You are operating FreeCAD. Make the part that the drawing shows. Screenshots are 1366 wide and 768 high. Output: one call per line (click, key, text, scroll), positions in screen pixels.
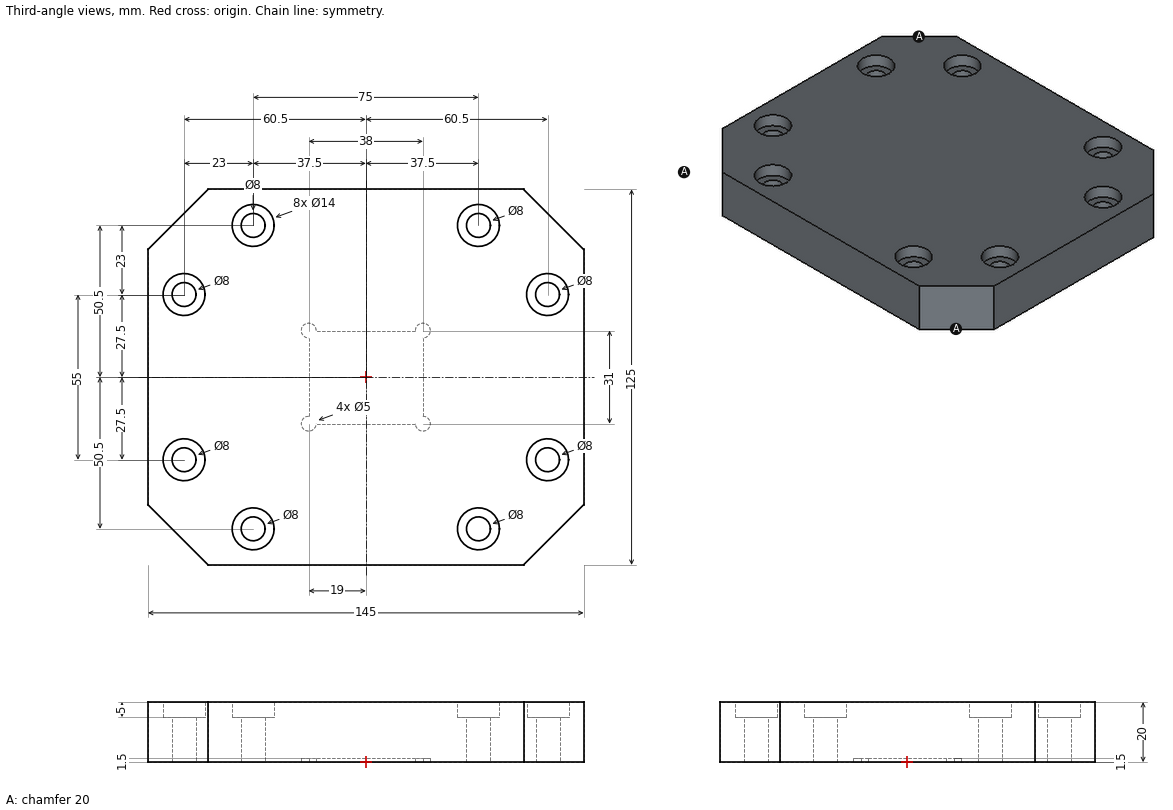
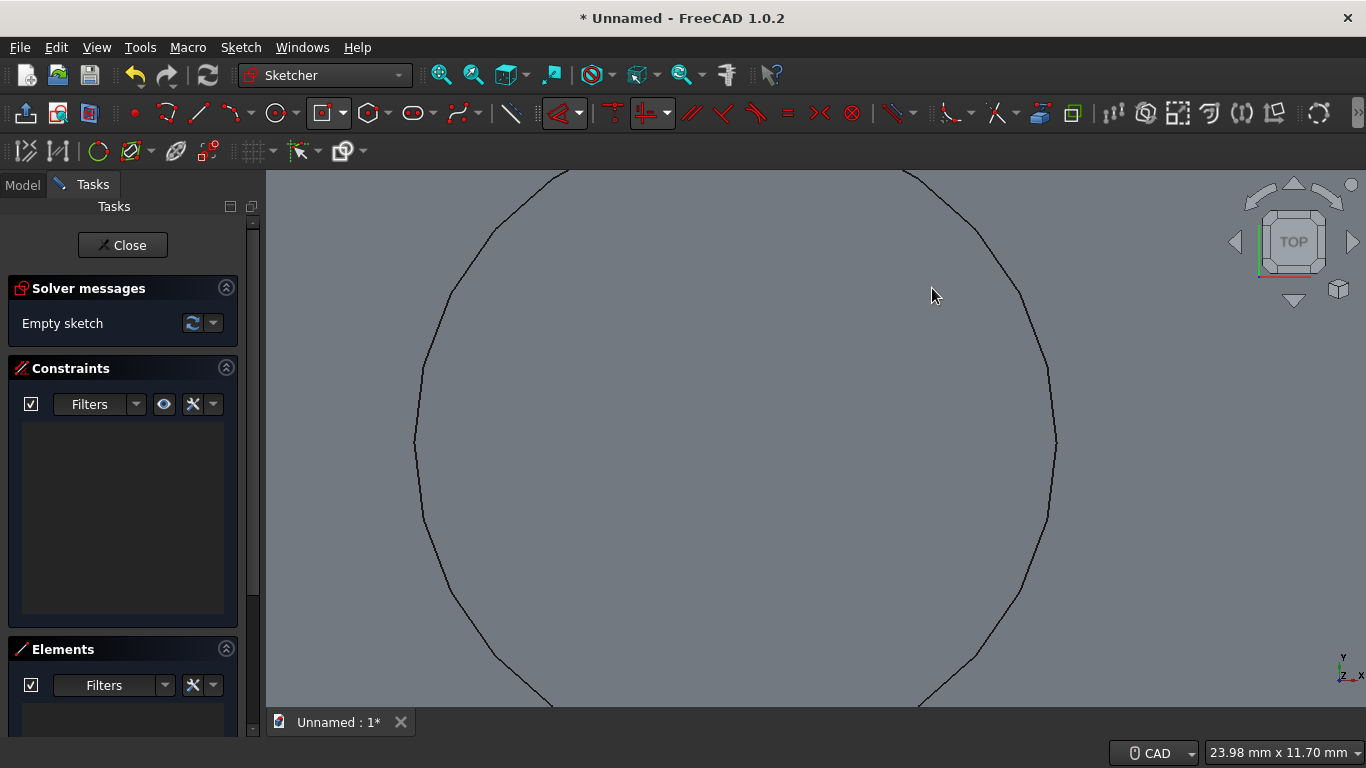
click(276, 114)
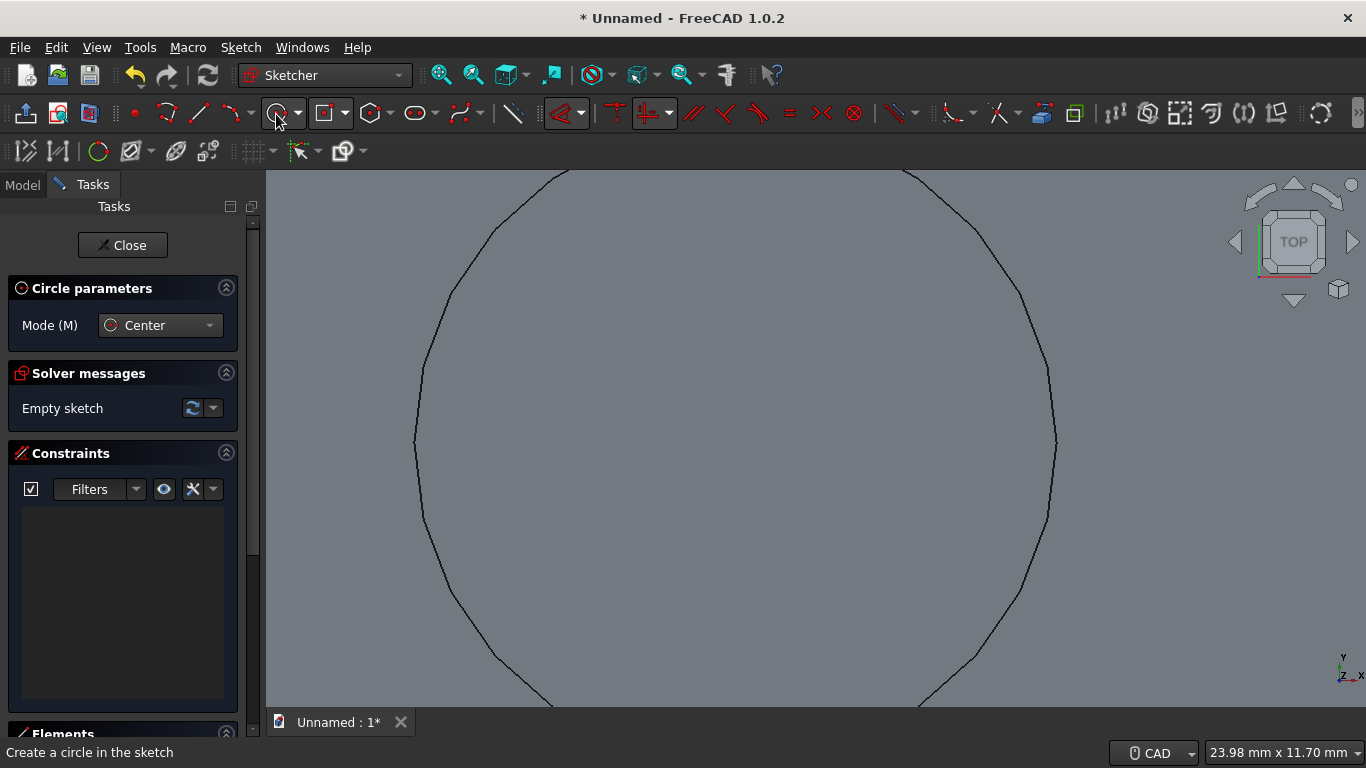
click(735, 443)
click(865, 313)
key(Escape)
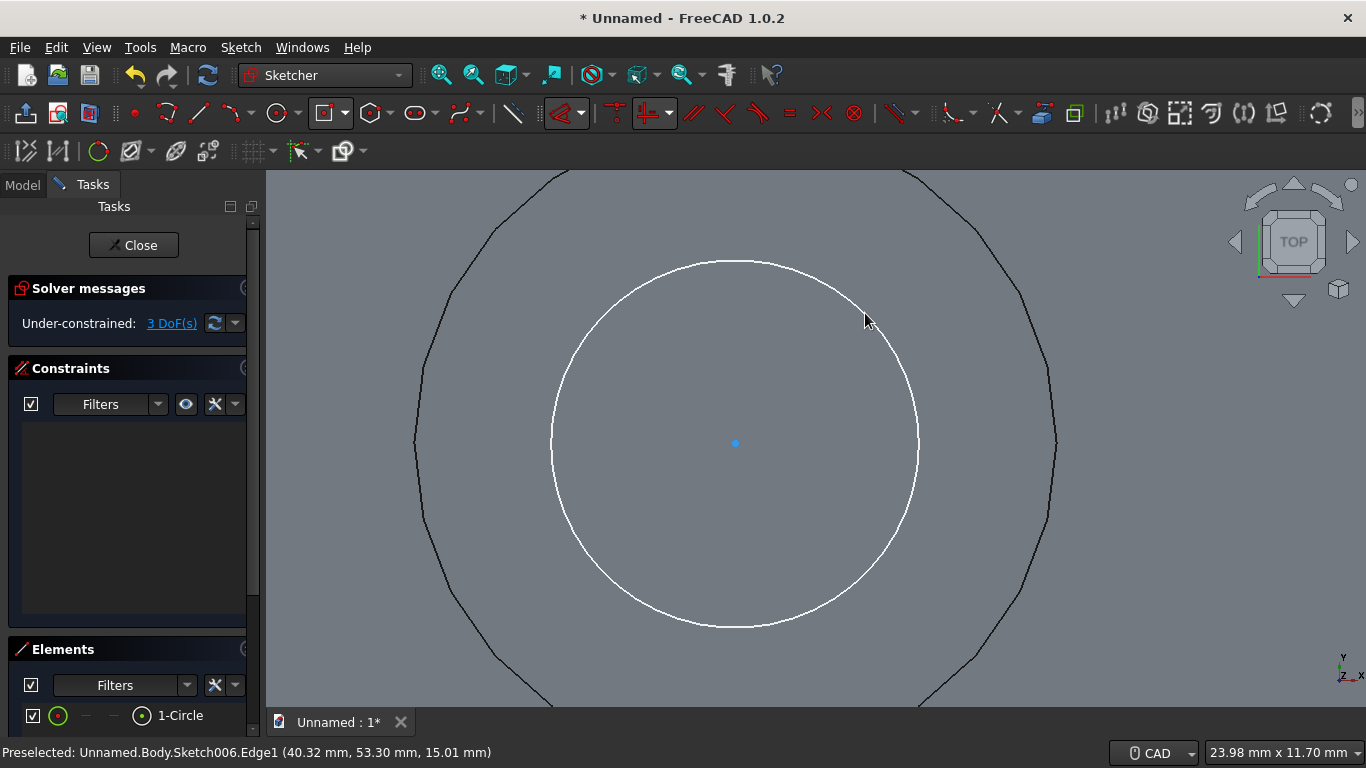
click(865, 314)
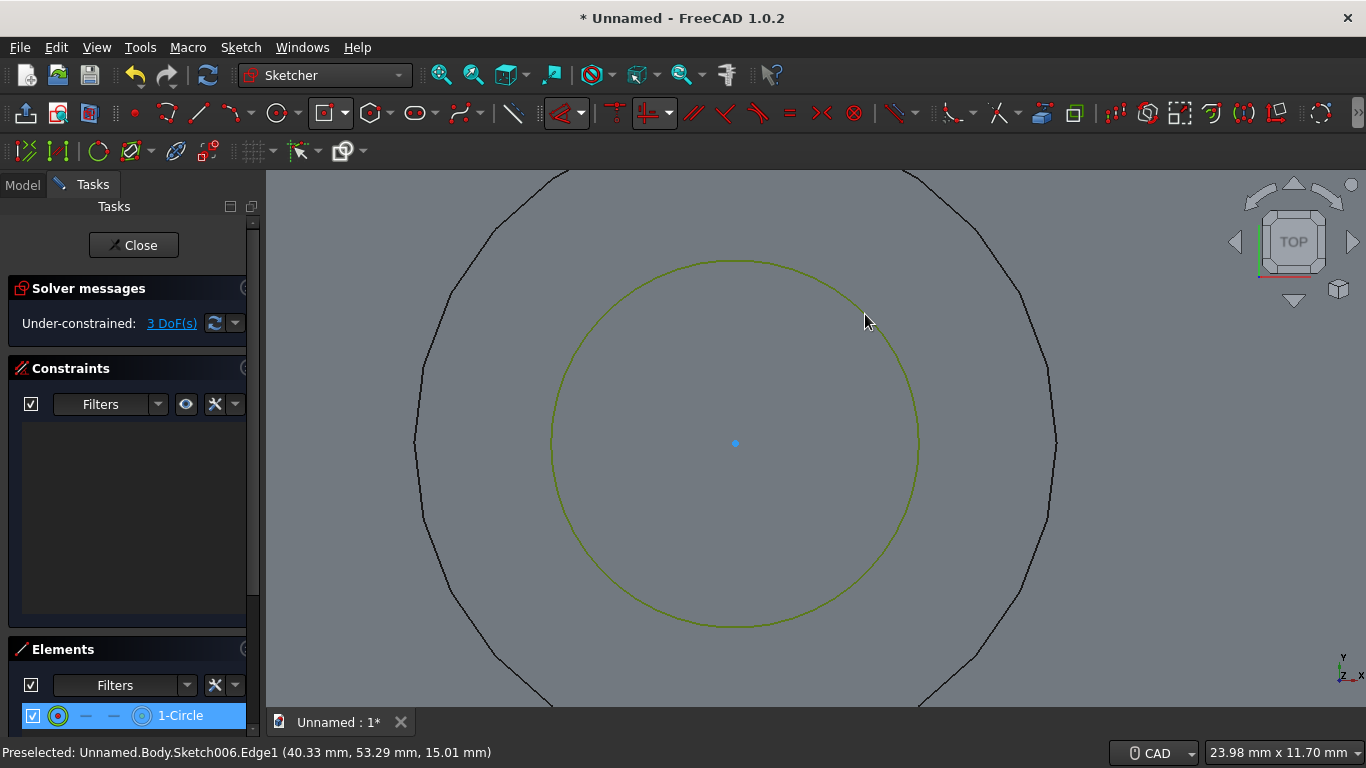
key(k)
key(o)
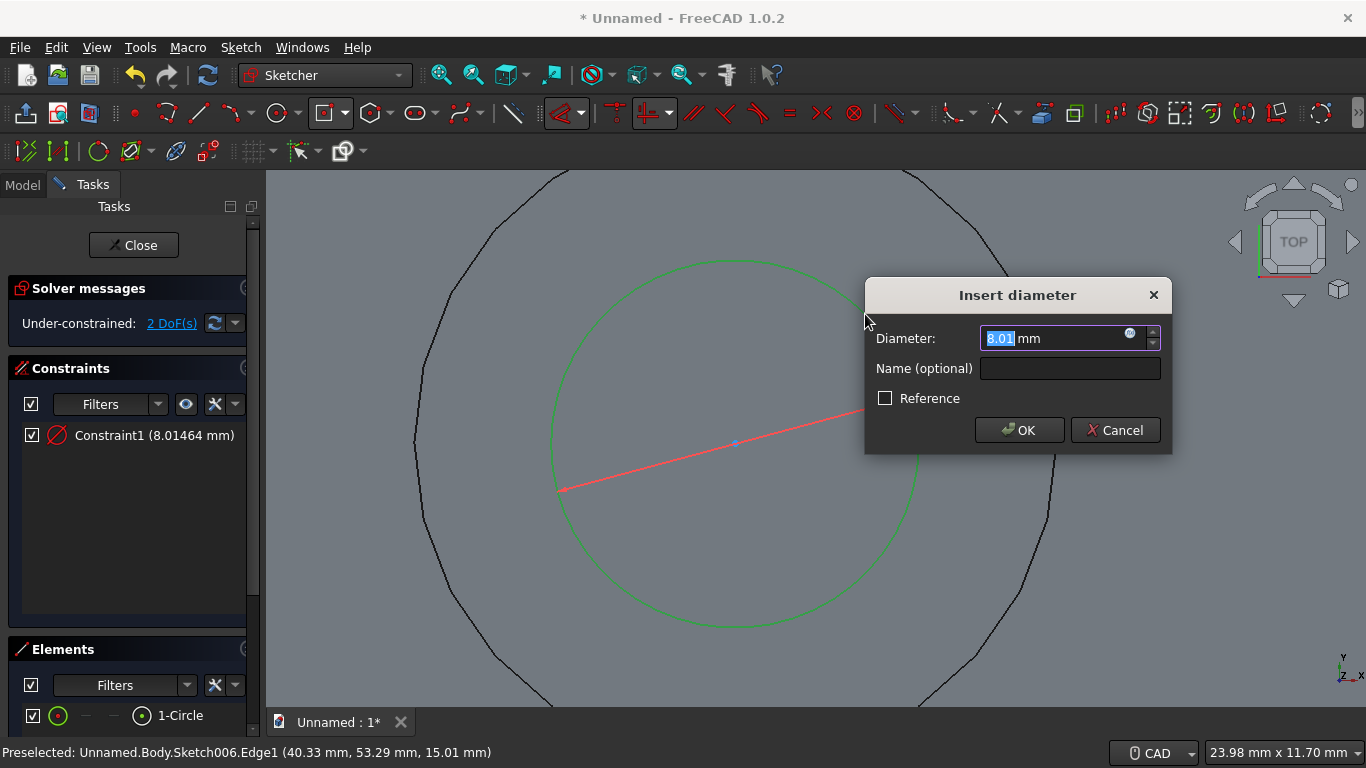
text(8)
key(Return)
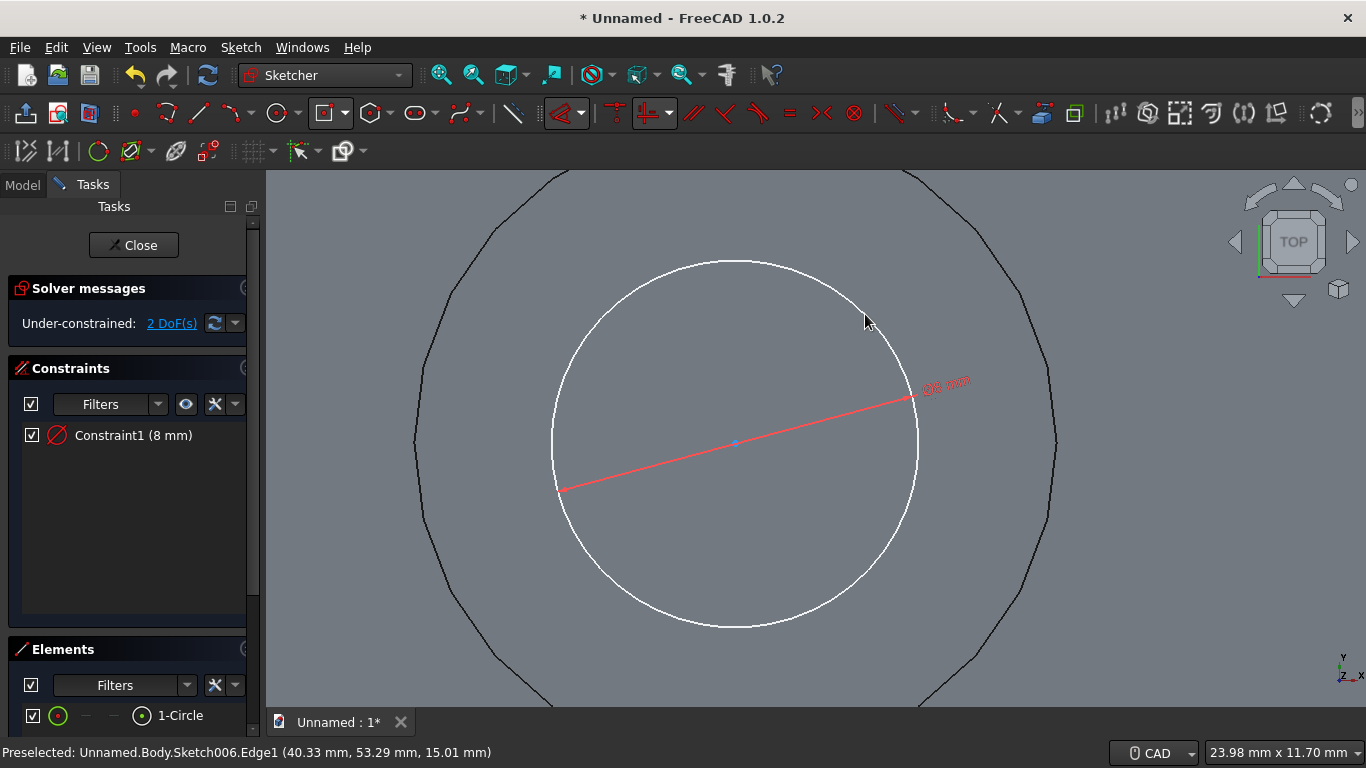
click(735, 444)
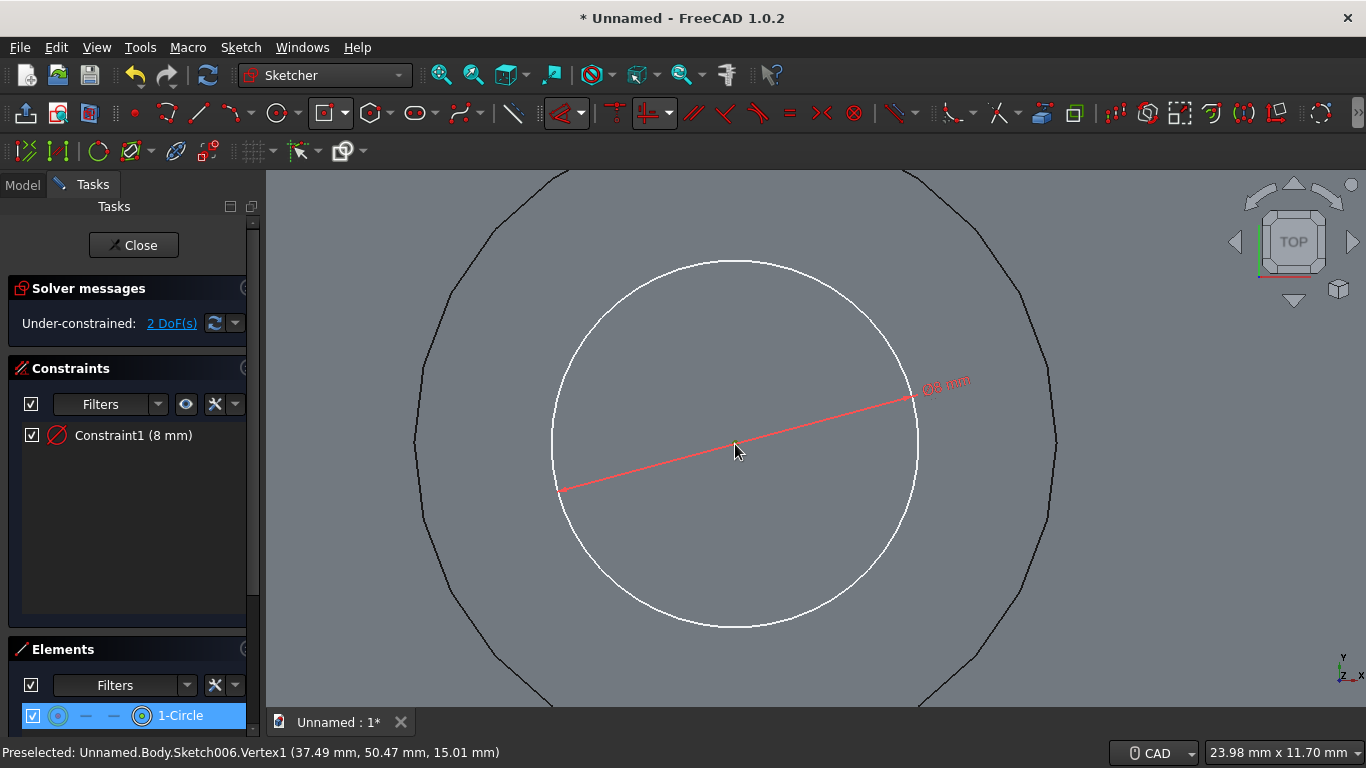
key(l)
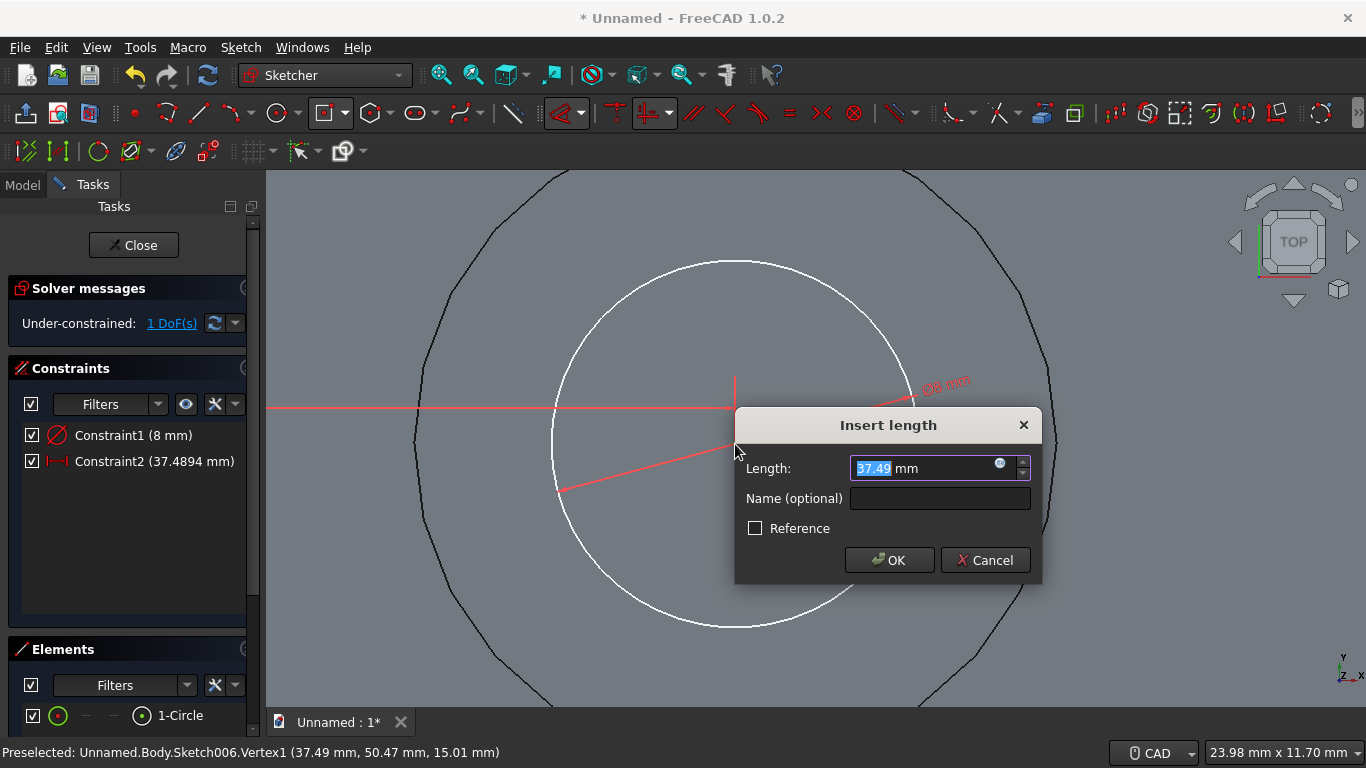
text(37.5)
key(Return)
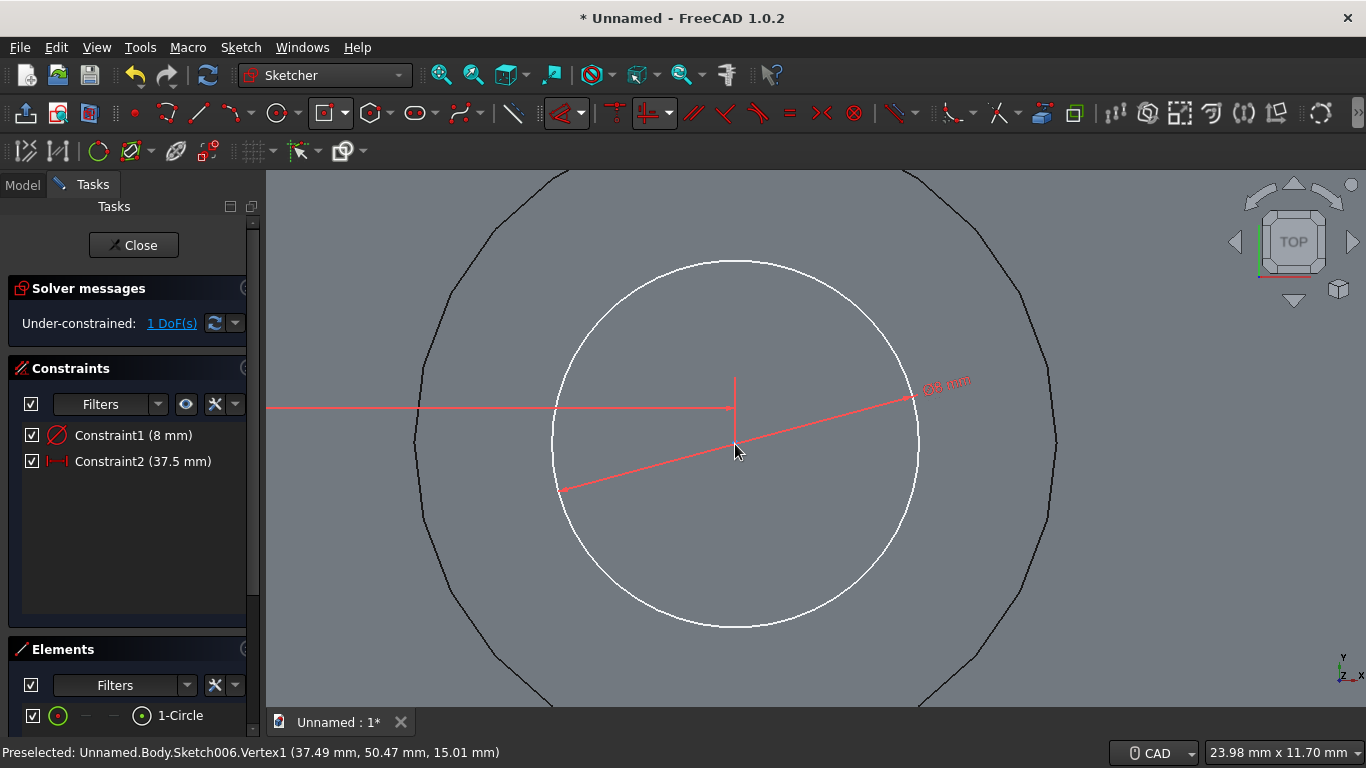
click(735, 444)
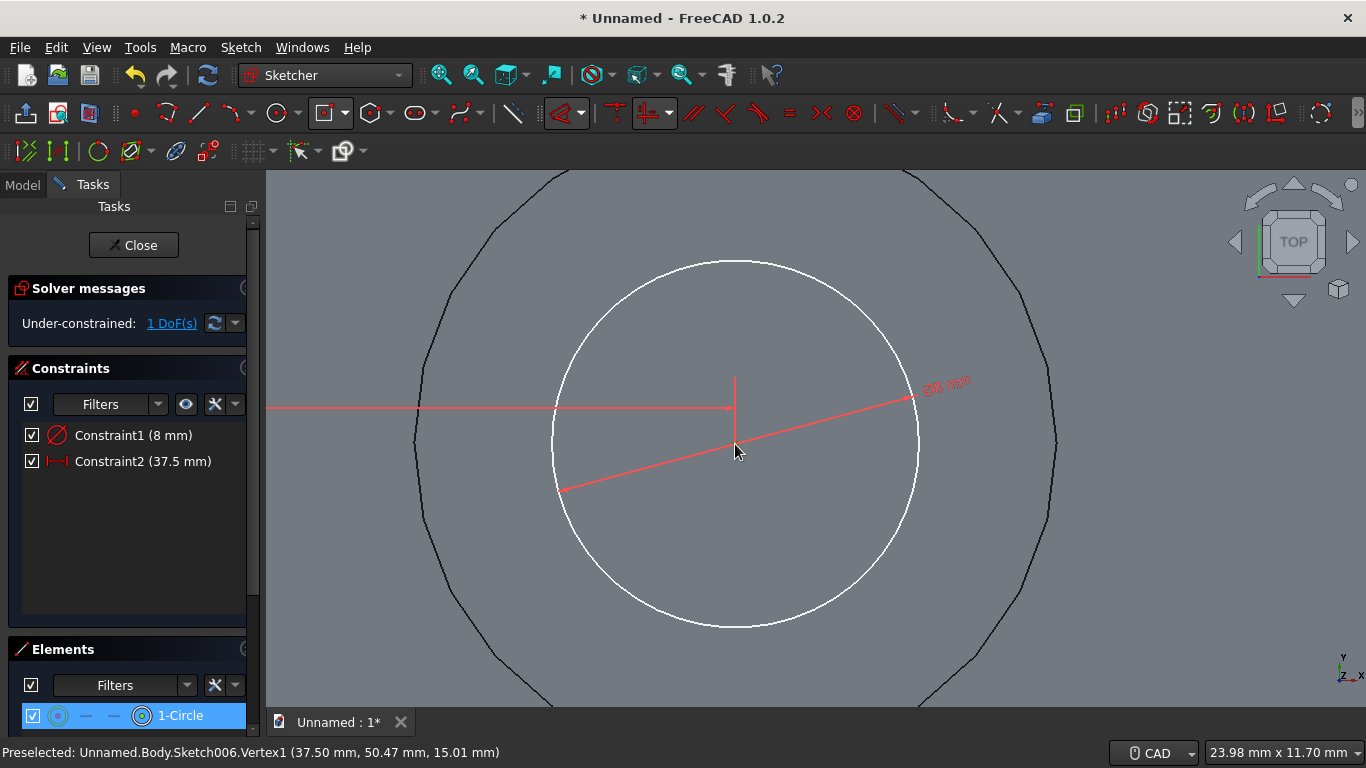
key(i)